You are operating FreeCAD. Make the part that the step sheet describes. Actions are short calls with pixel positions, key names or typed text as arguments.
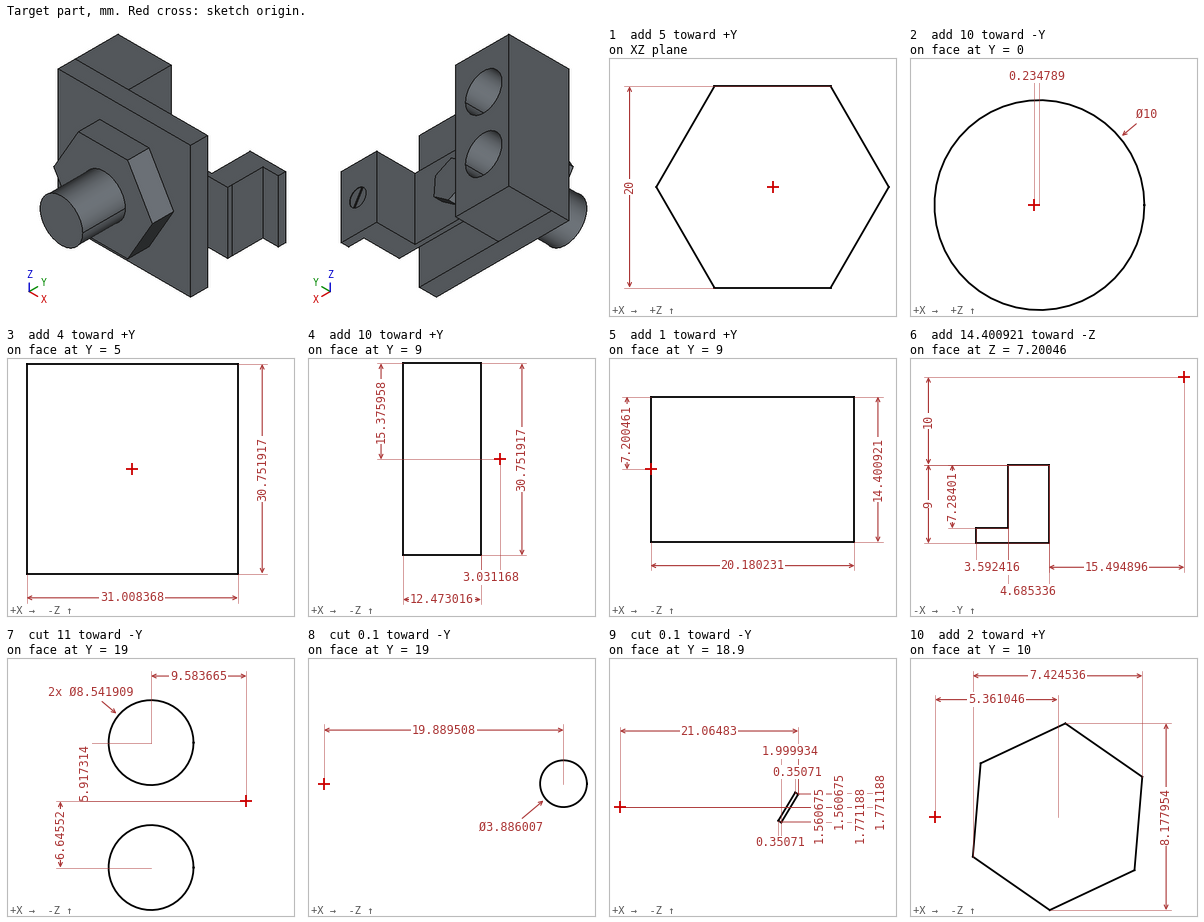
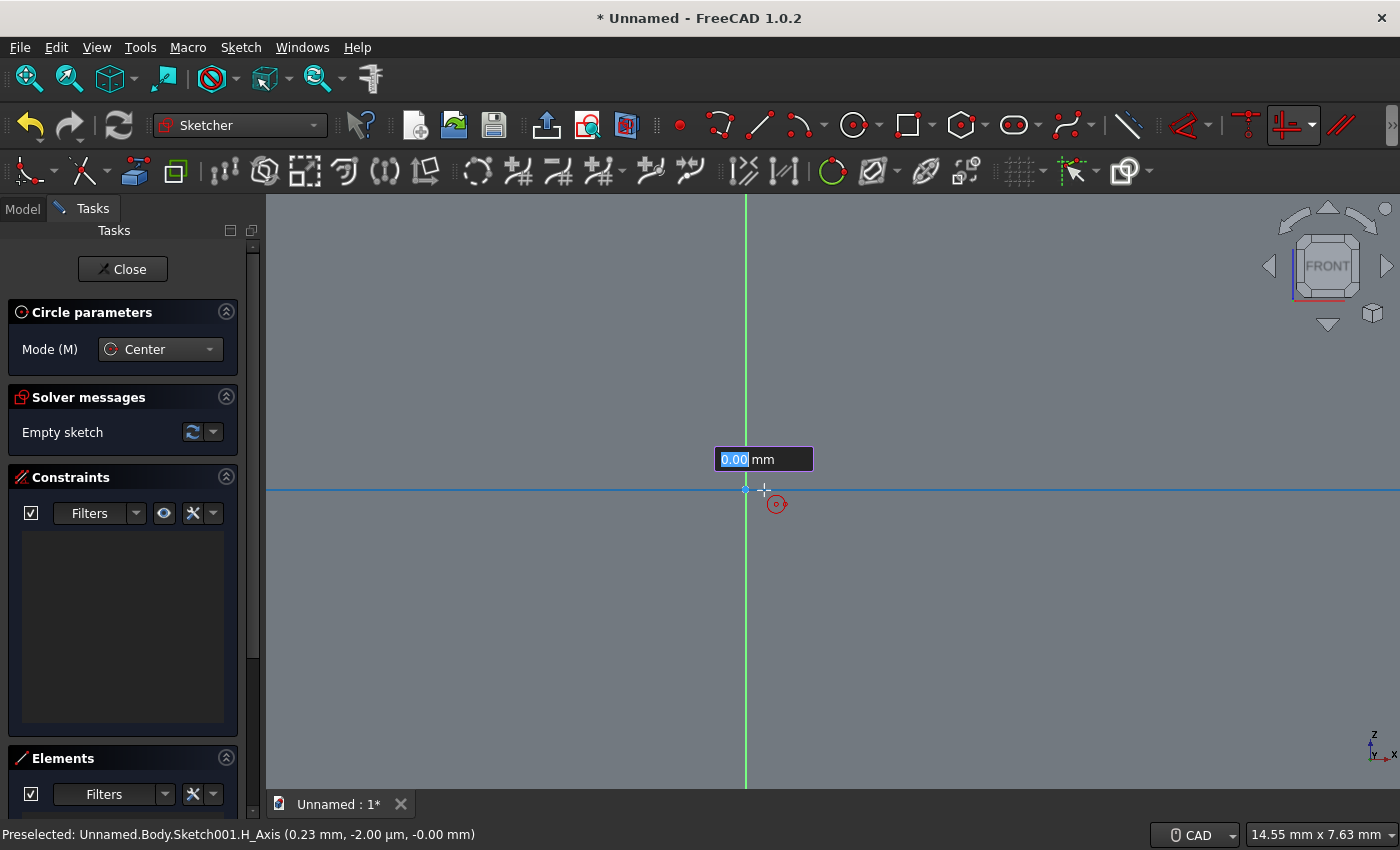
scroll(765, 493, down, 4)
move(889, 368)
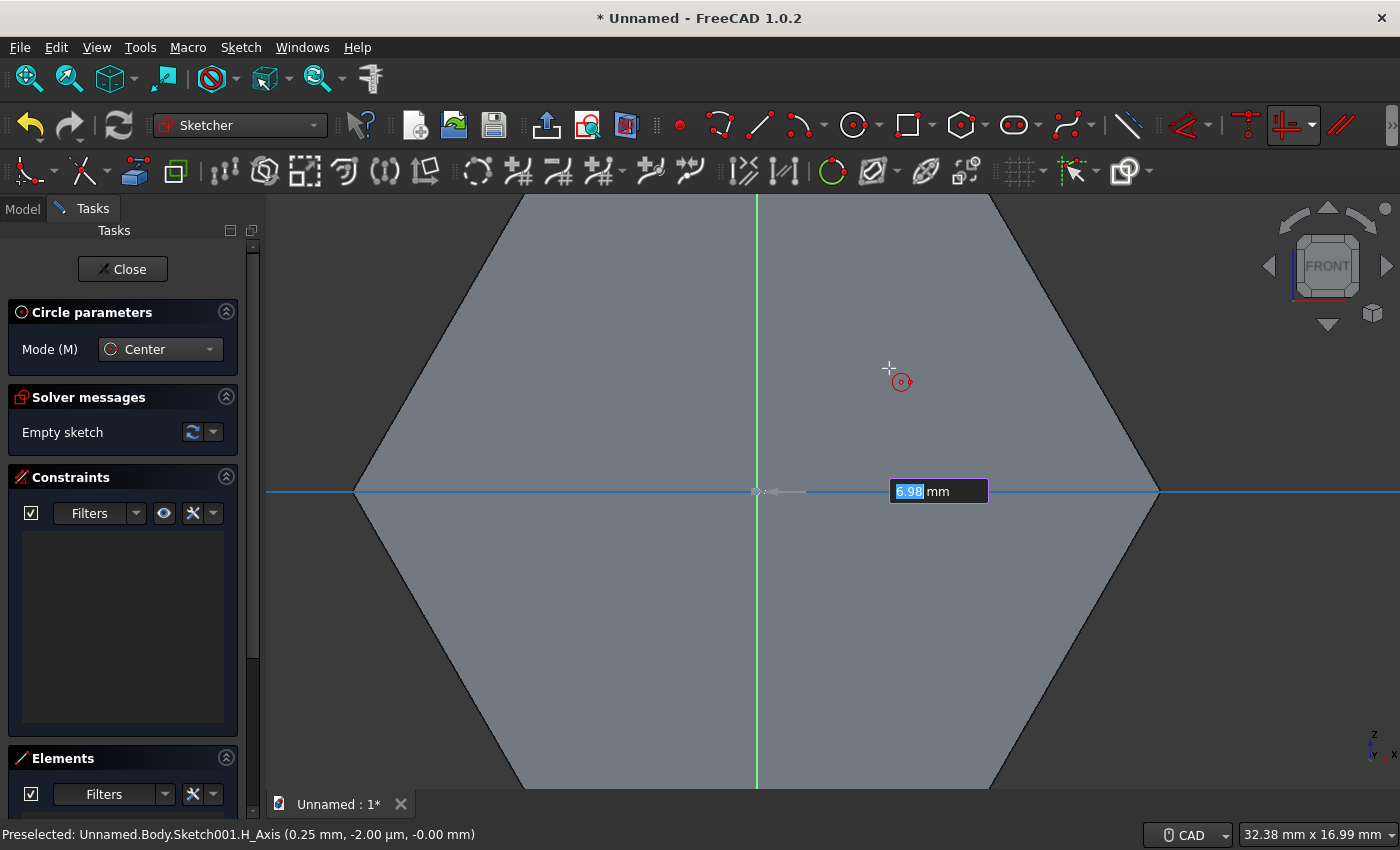
text(10)
key(Return)
key(Escape)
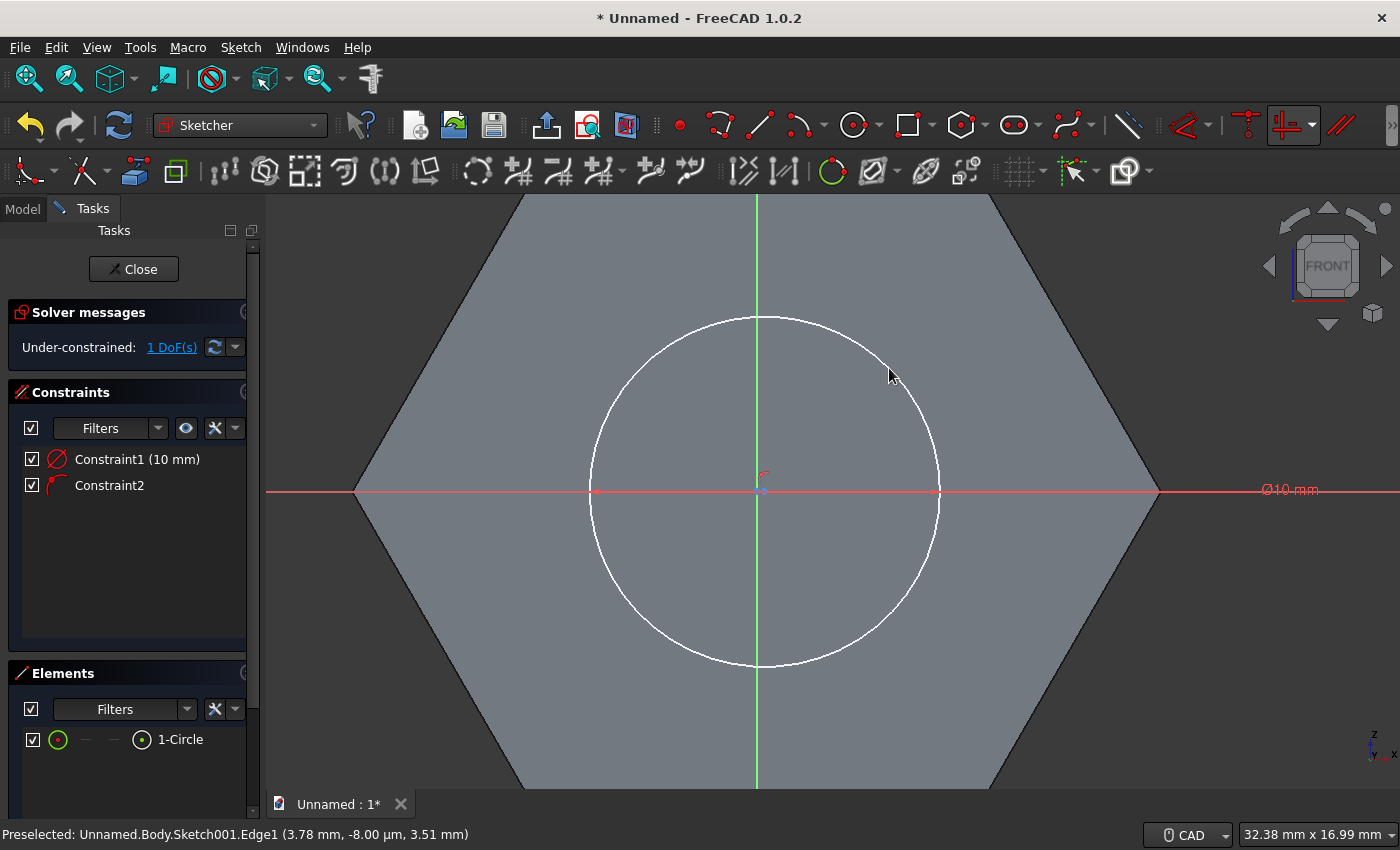
click(1184, 126)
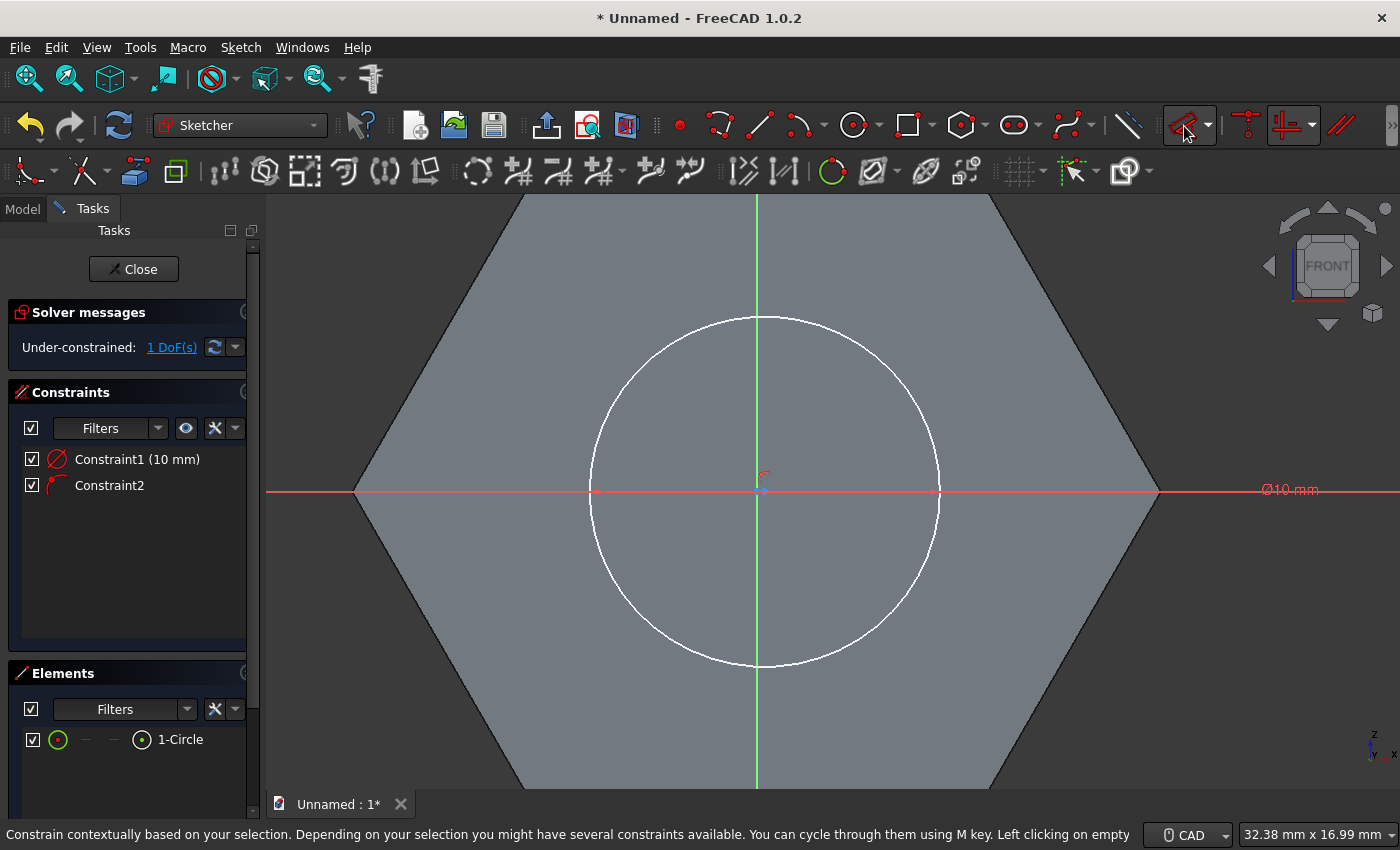
scroll(765, 492, up, 8)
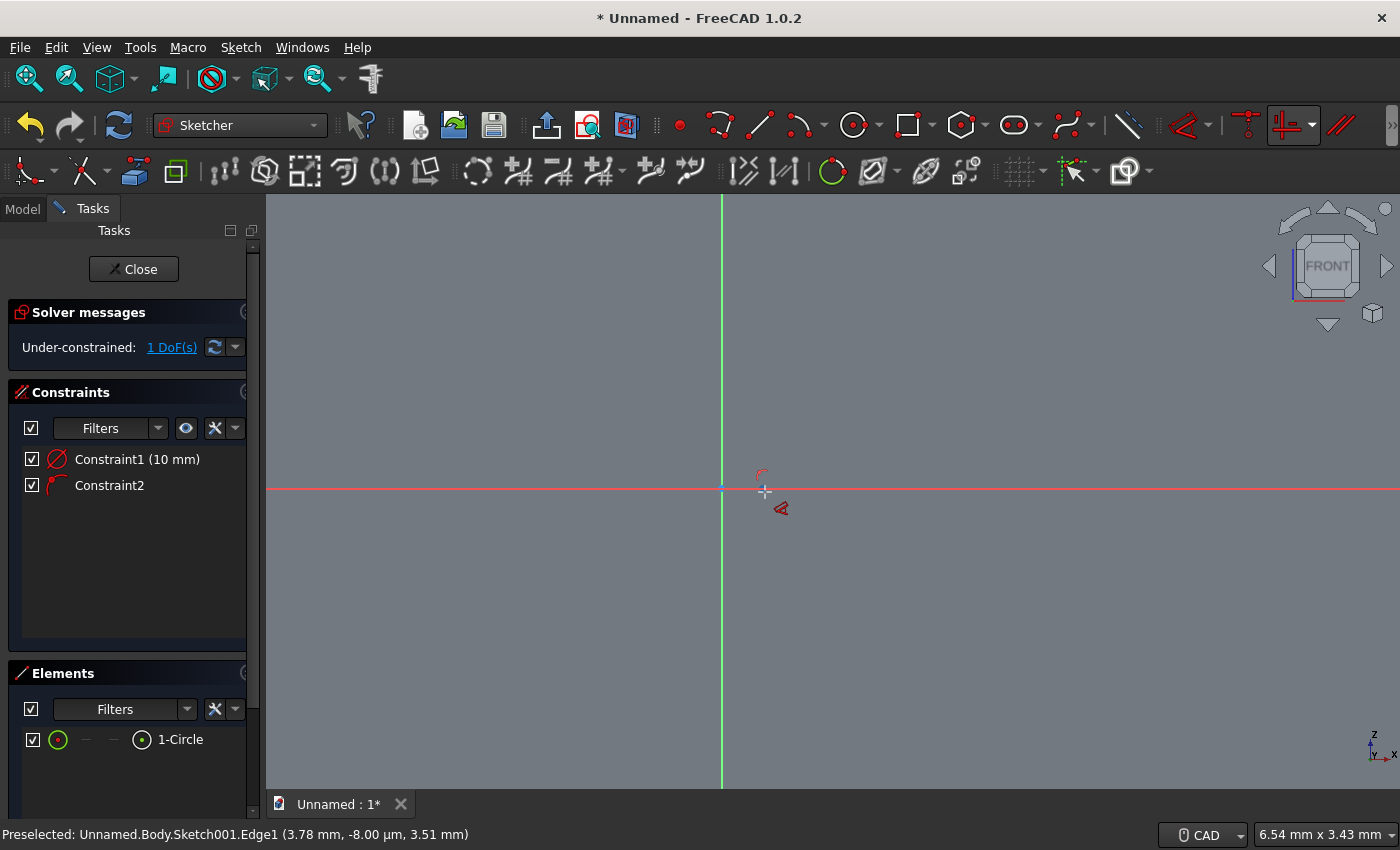
click(762, 489)
click(742, 523)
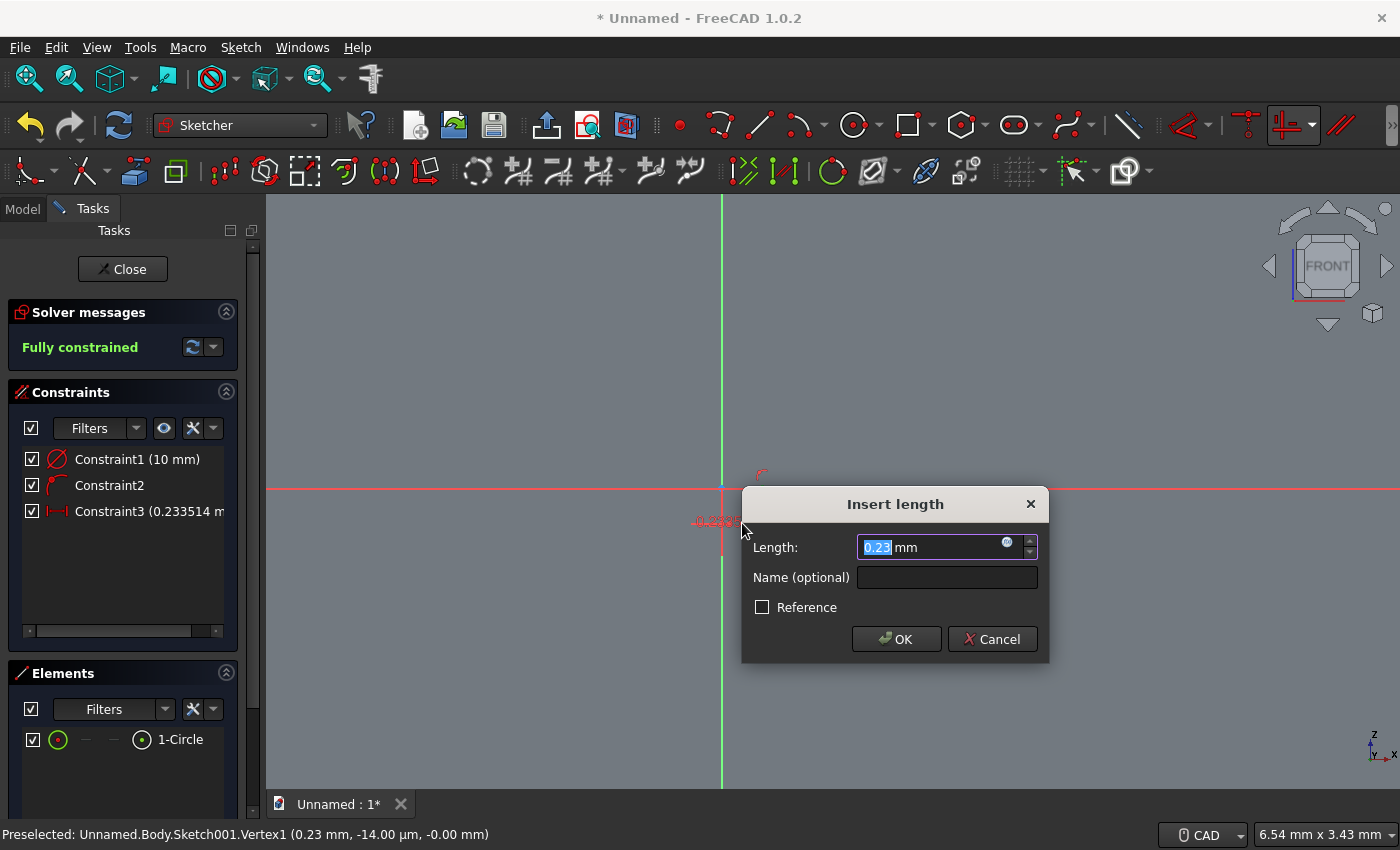
text(0.234789)
key(Return)
key(Escape)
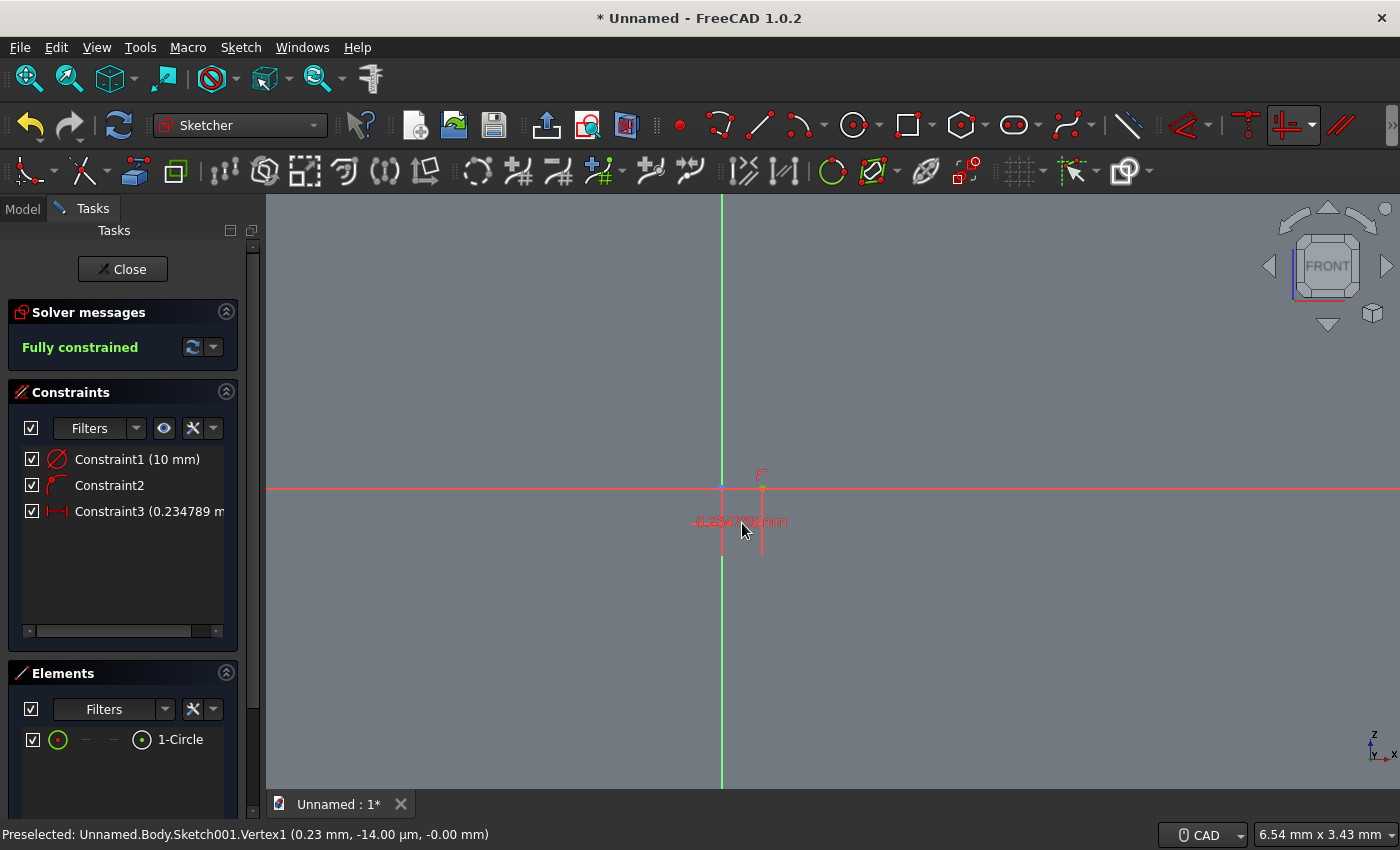
click(123, 269)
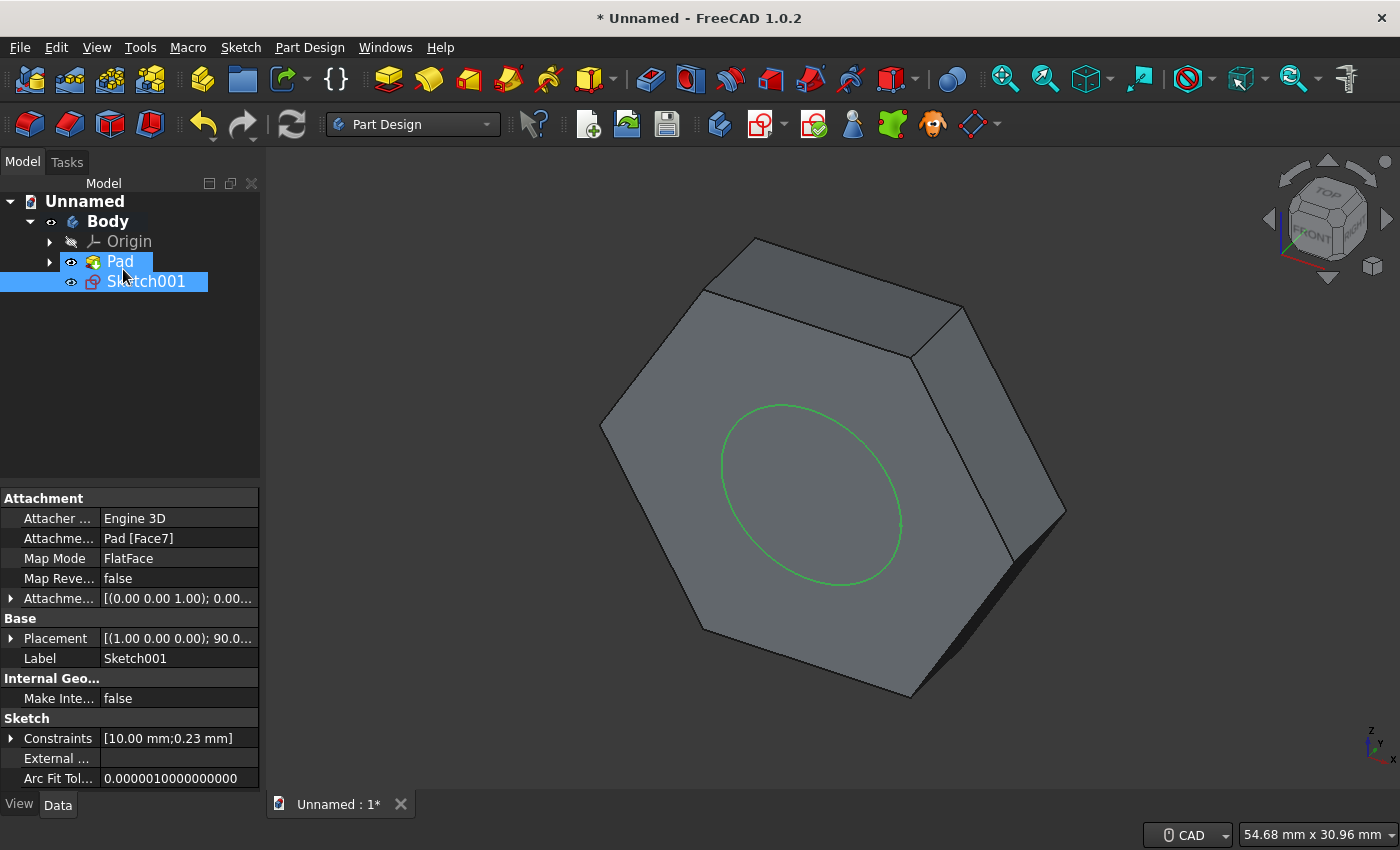
click(390, 80)